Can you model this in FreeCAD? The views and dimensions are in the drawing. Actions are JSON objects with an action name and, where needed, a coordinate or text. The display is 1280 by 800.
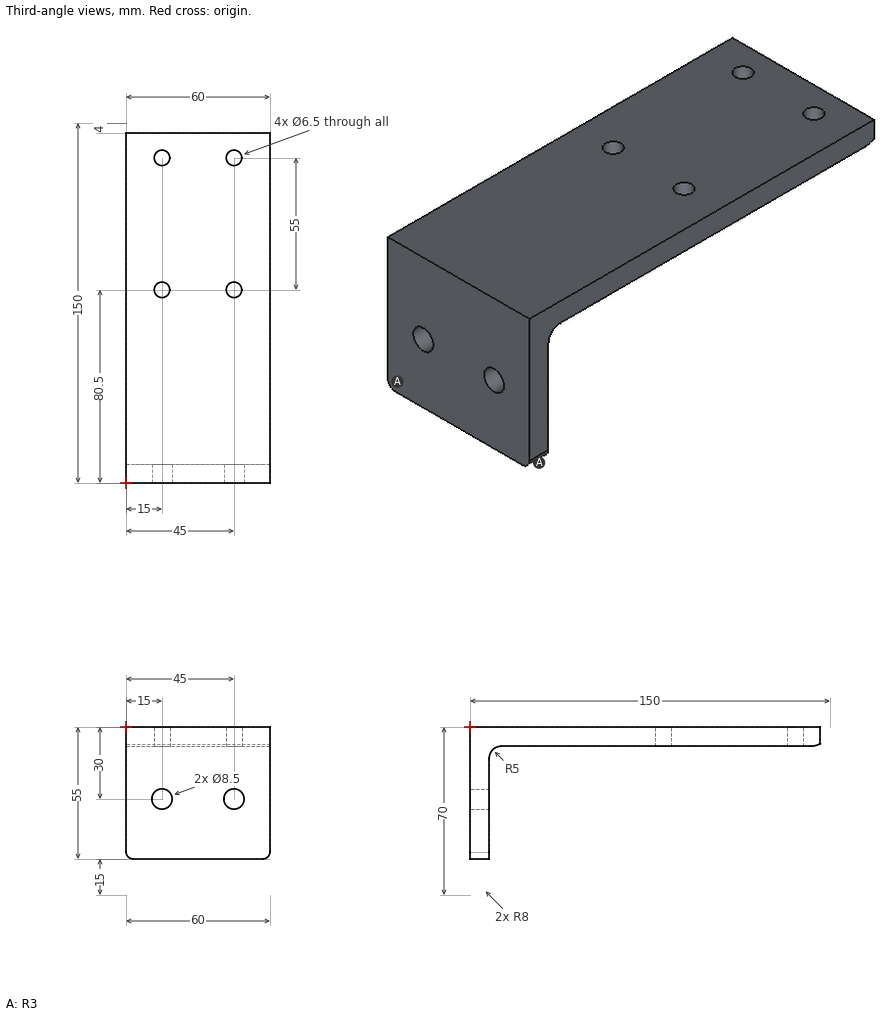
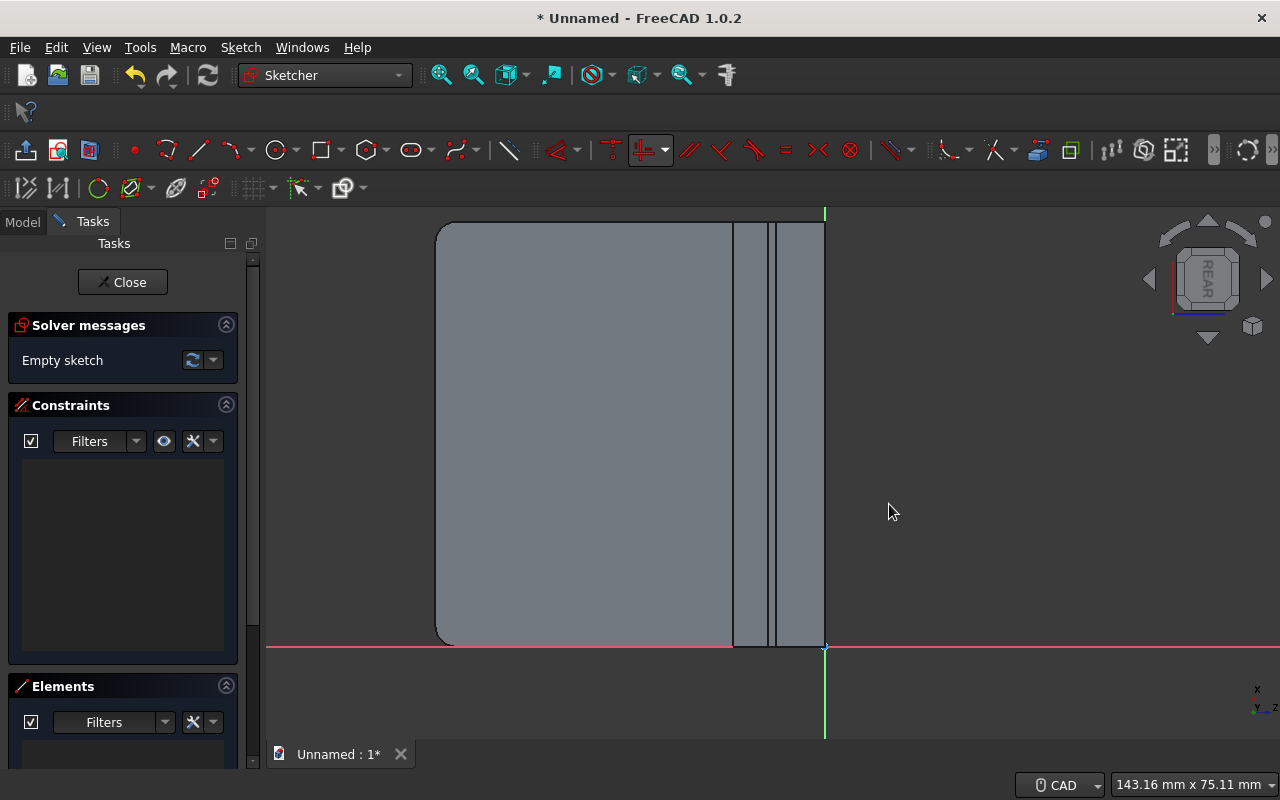
{"action": "key", "text": "g c"}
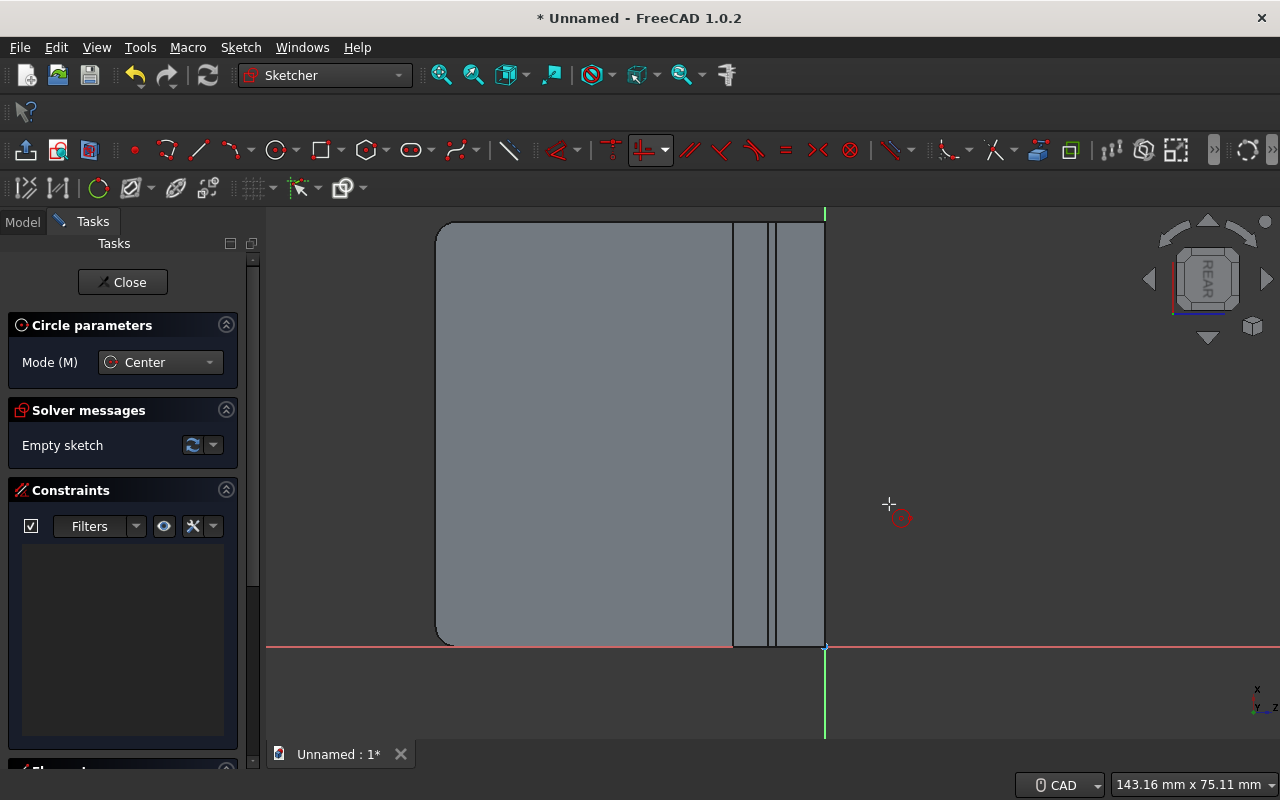
{"action": "left_click", "coordinate": [612, 541]}
{"action": "left_click", "coordinate": [634, 519]}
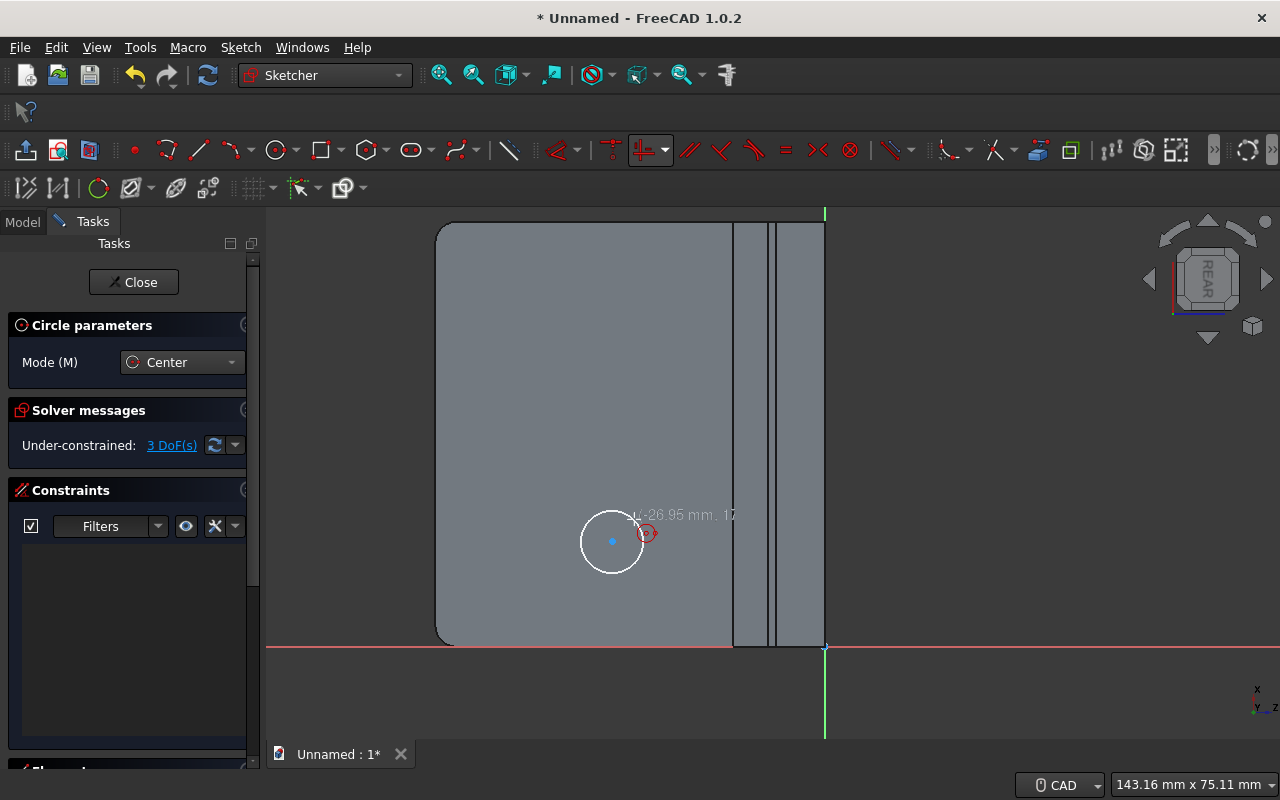
{"action": "left_click", "coordinate": [612, 328]}
{"action": "left_click", "coordinate": [634, 307]}
{"action": "key", "text": "Escape"}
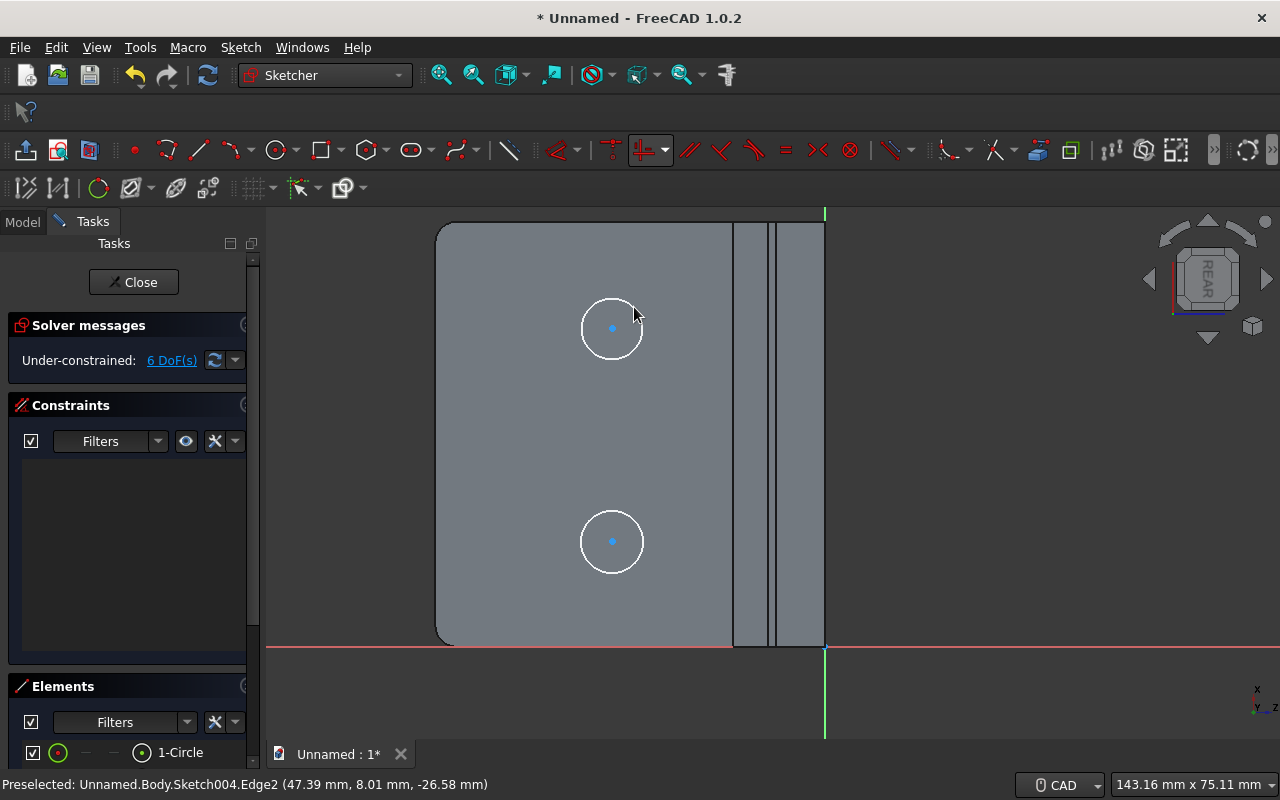
{"action": "left_click", "coordinate": [634, 520]}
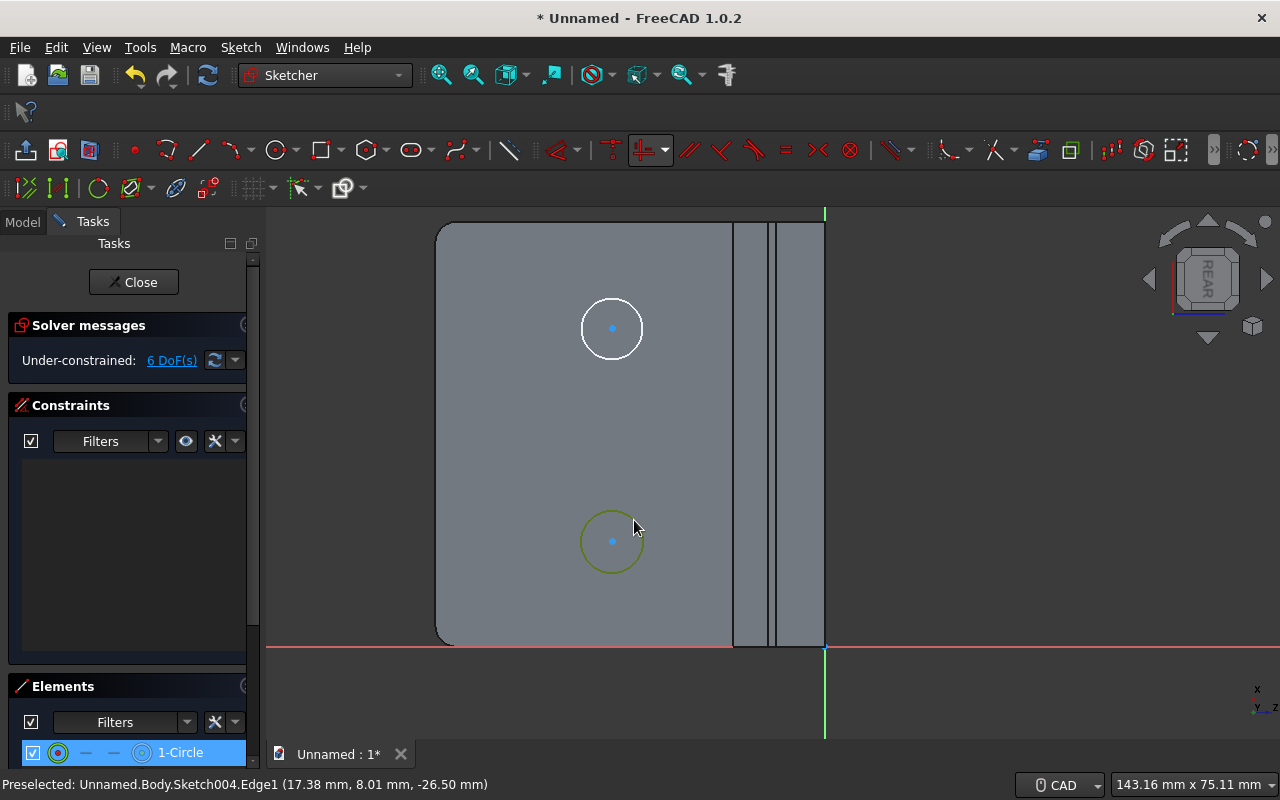
{"action": "left_click", "coordinate": [633, 307]}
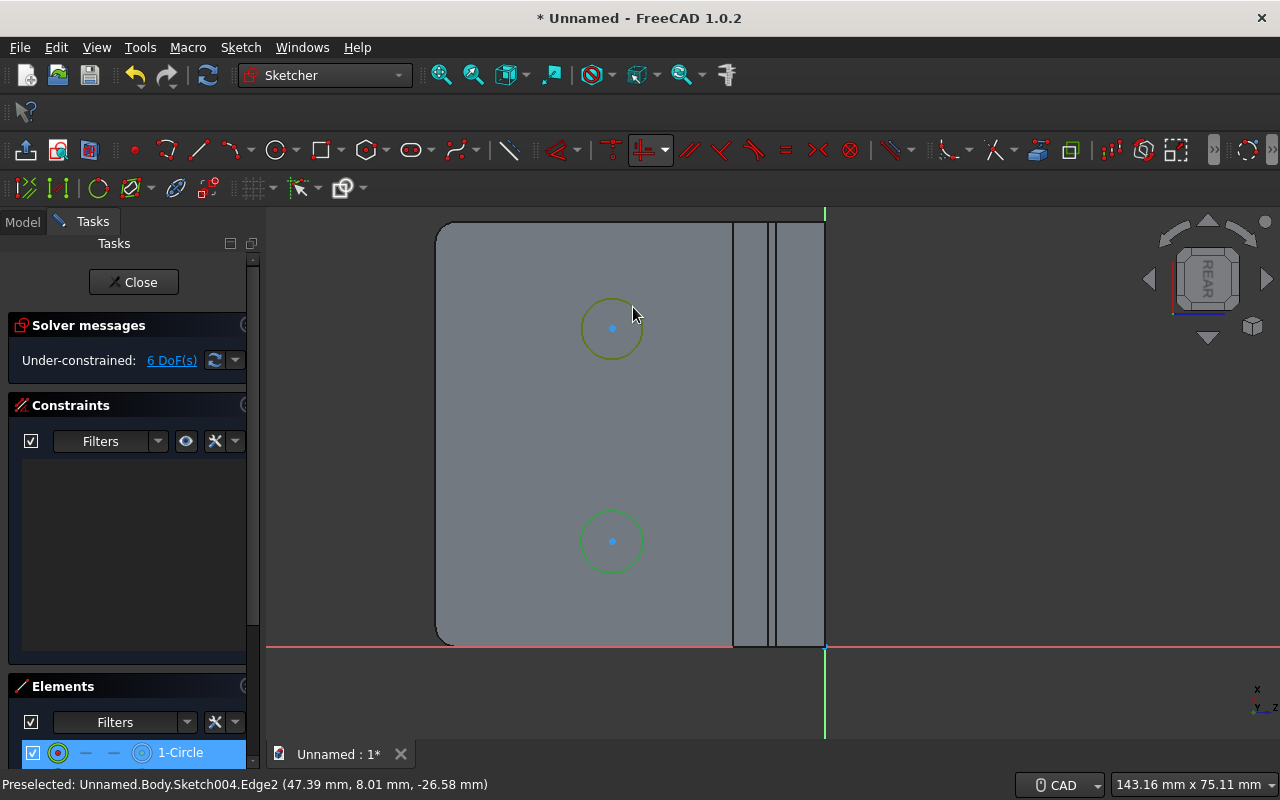
{"action": "key", "text": "e"}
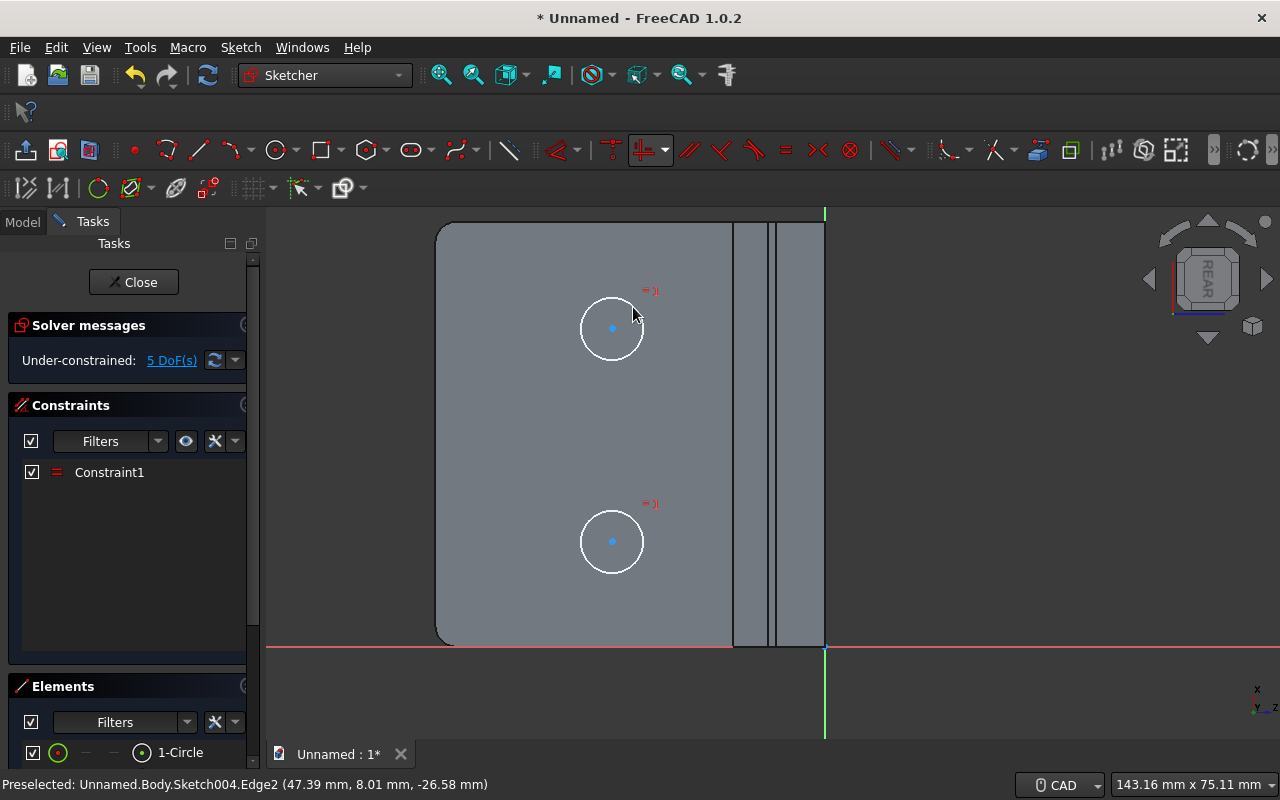
{"action": "key", "text": "d"}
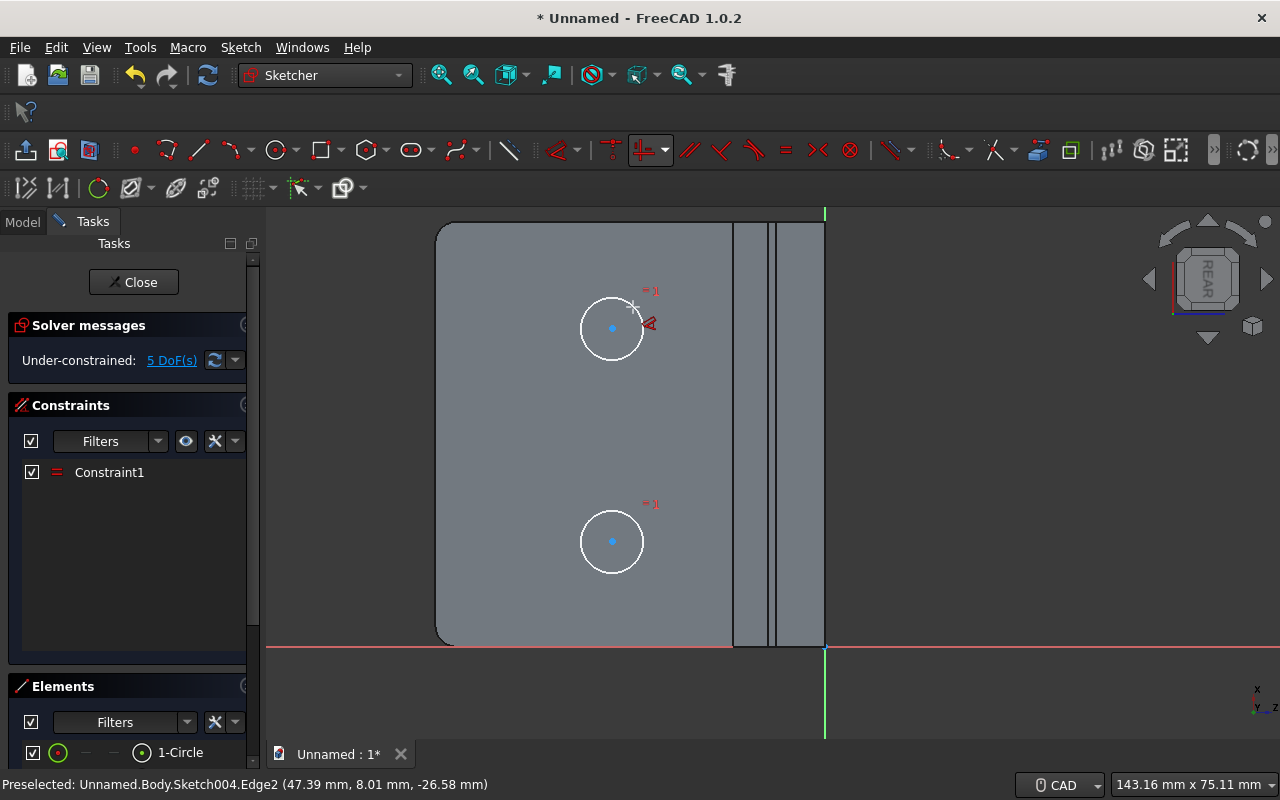
{"action": "left_click", "coordinate": [634, 520]}
{"action": "left_click", "coordinate": [657, 497]}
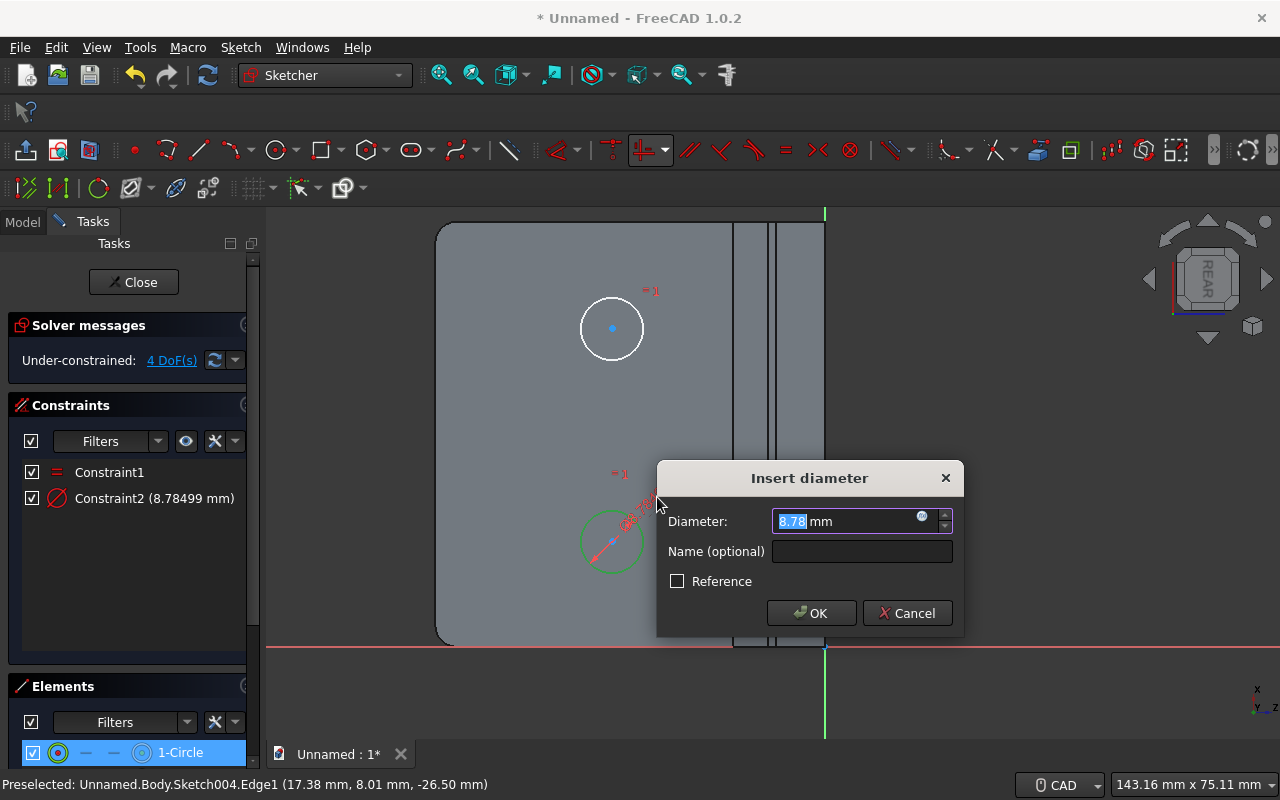
{"action": "type", "text": "8.5"}
{"action": "key", "text": "Return"}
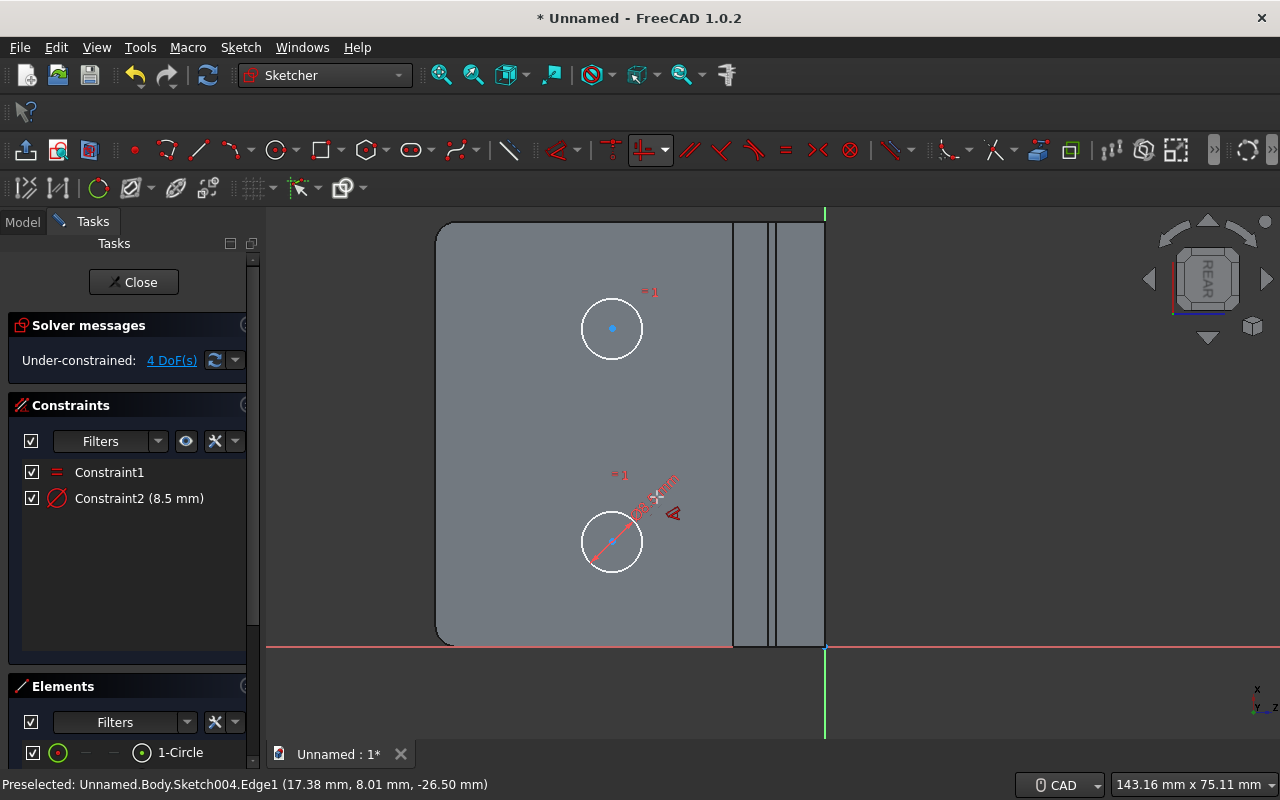
{"action": "left_click", "coordinate": [612, 542]}
{"action": "left_click", "coordinate": [718, 681]}